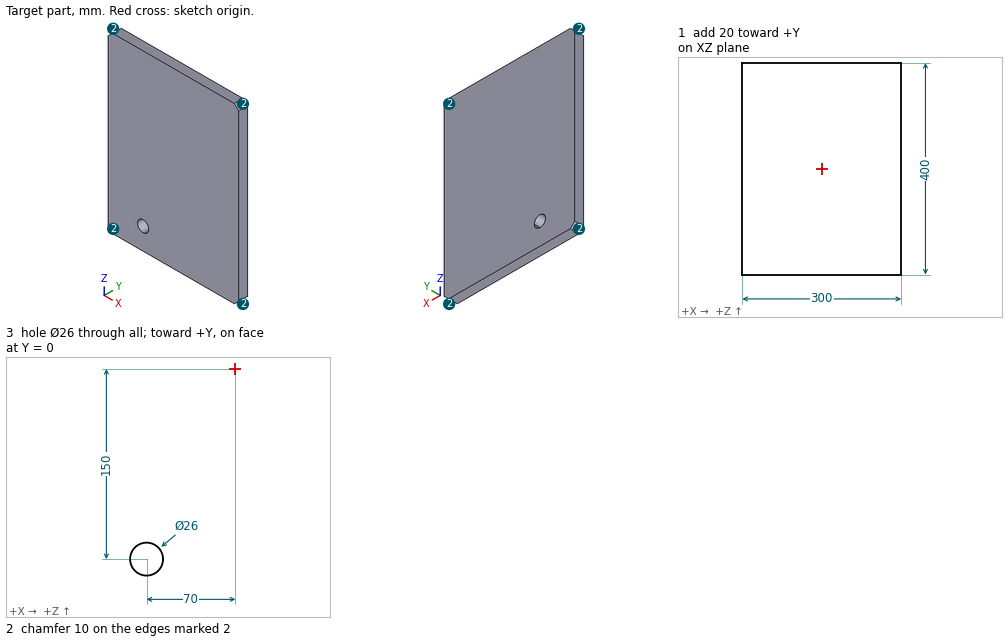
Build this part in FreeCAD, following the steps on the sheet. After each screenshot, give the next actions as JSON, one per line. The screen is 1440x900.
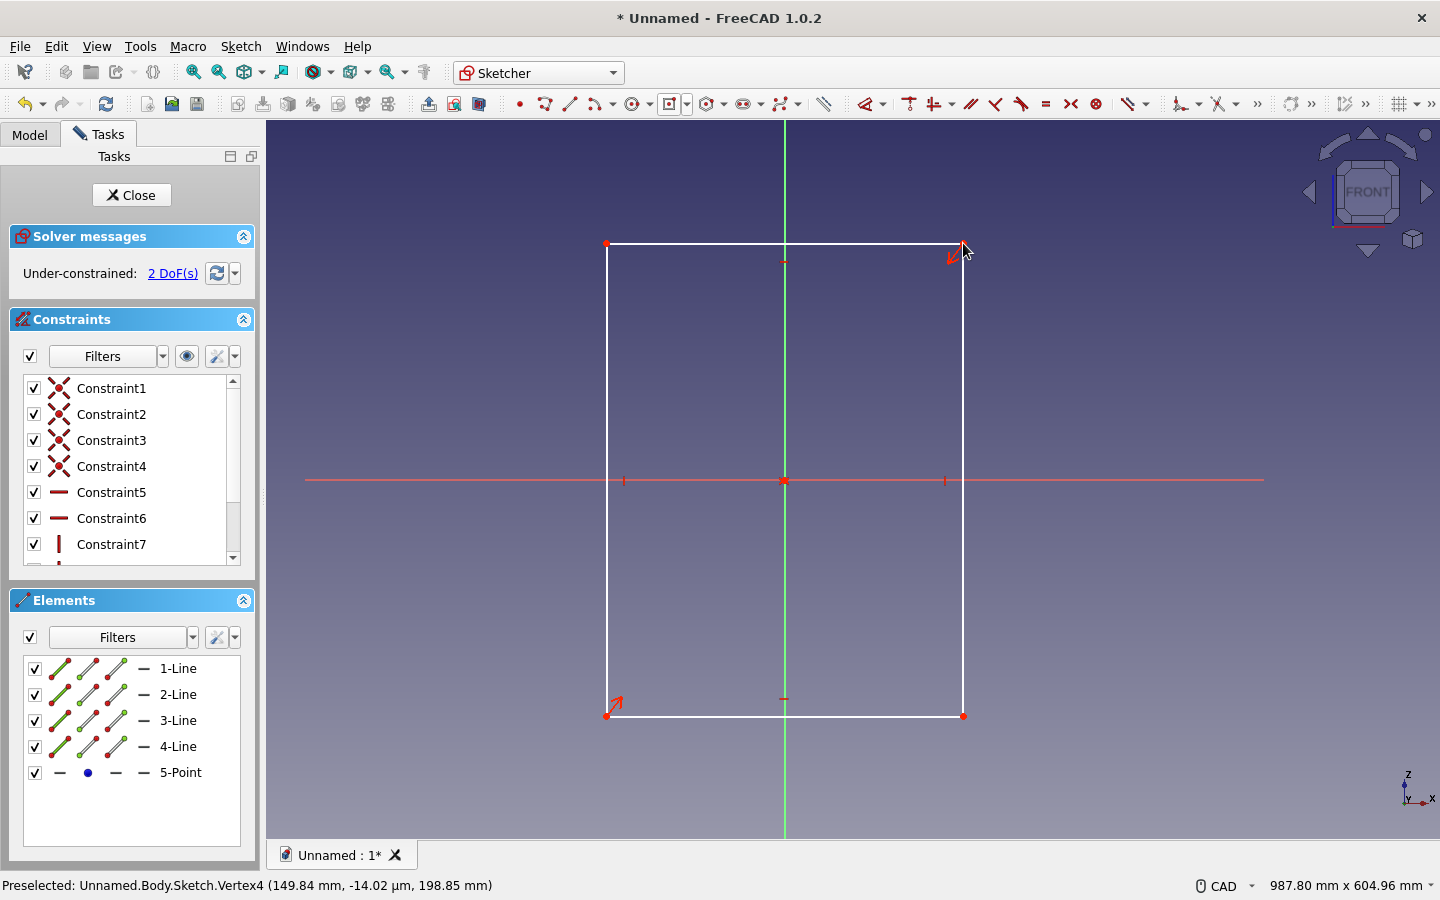
{"action": "left_click", "coordinate": [864, 104]}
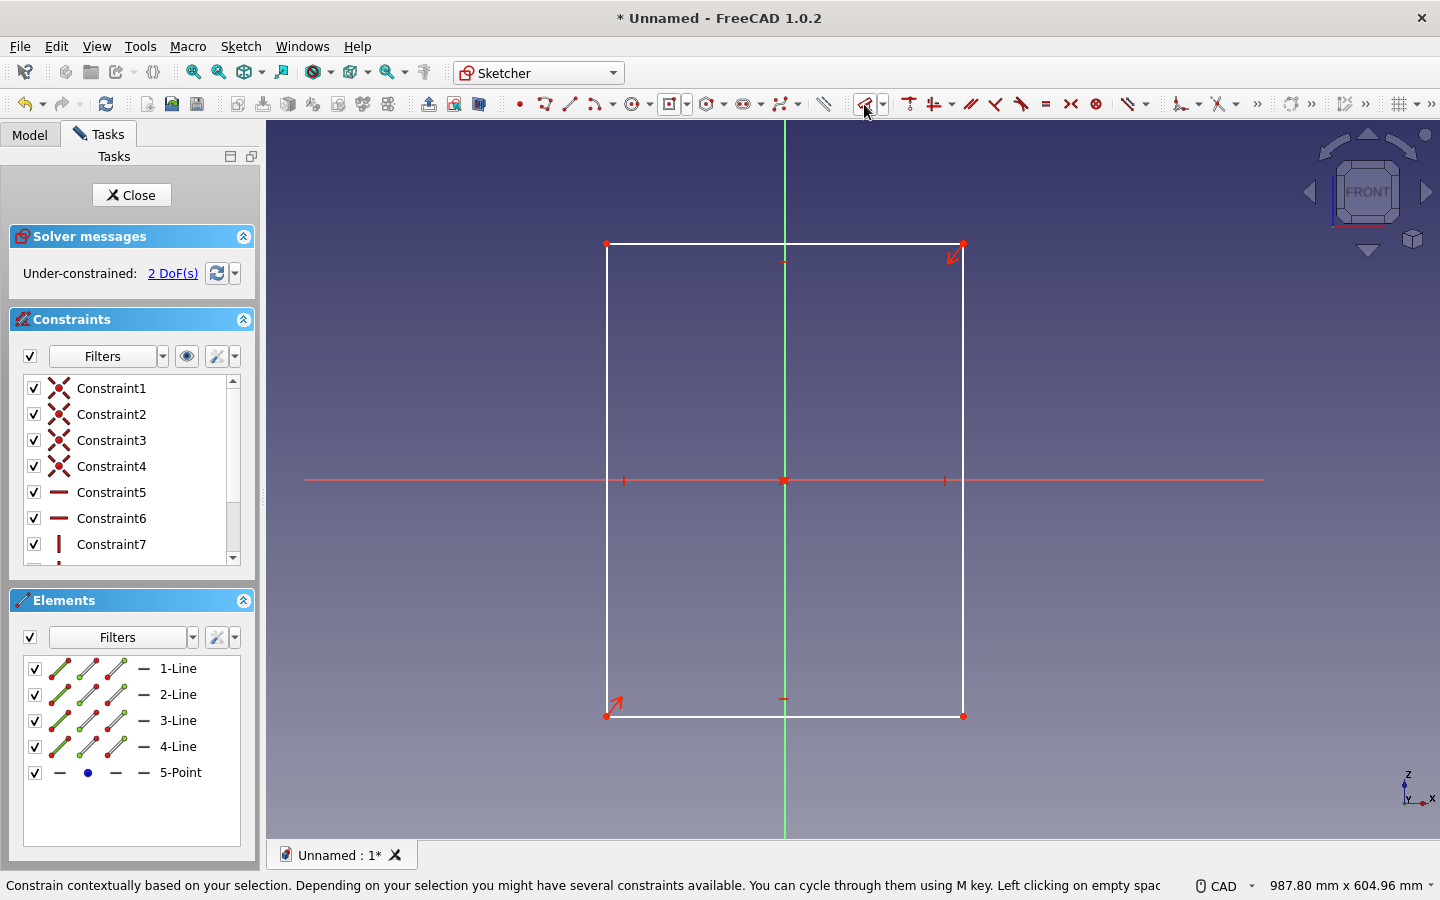
{"action": "left_click", "coordinate": [714, 717]}
{"action": "left_click", "coordinate": [703, 751]}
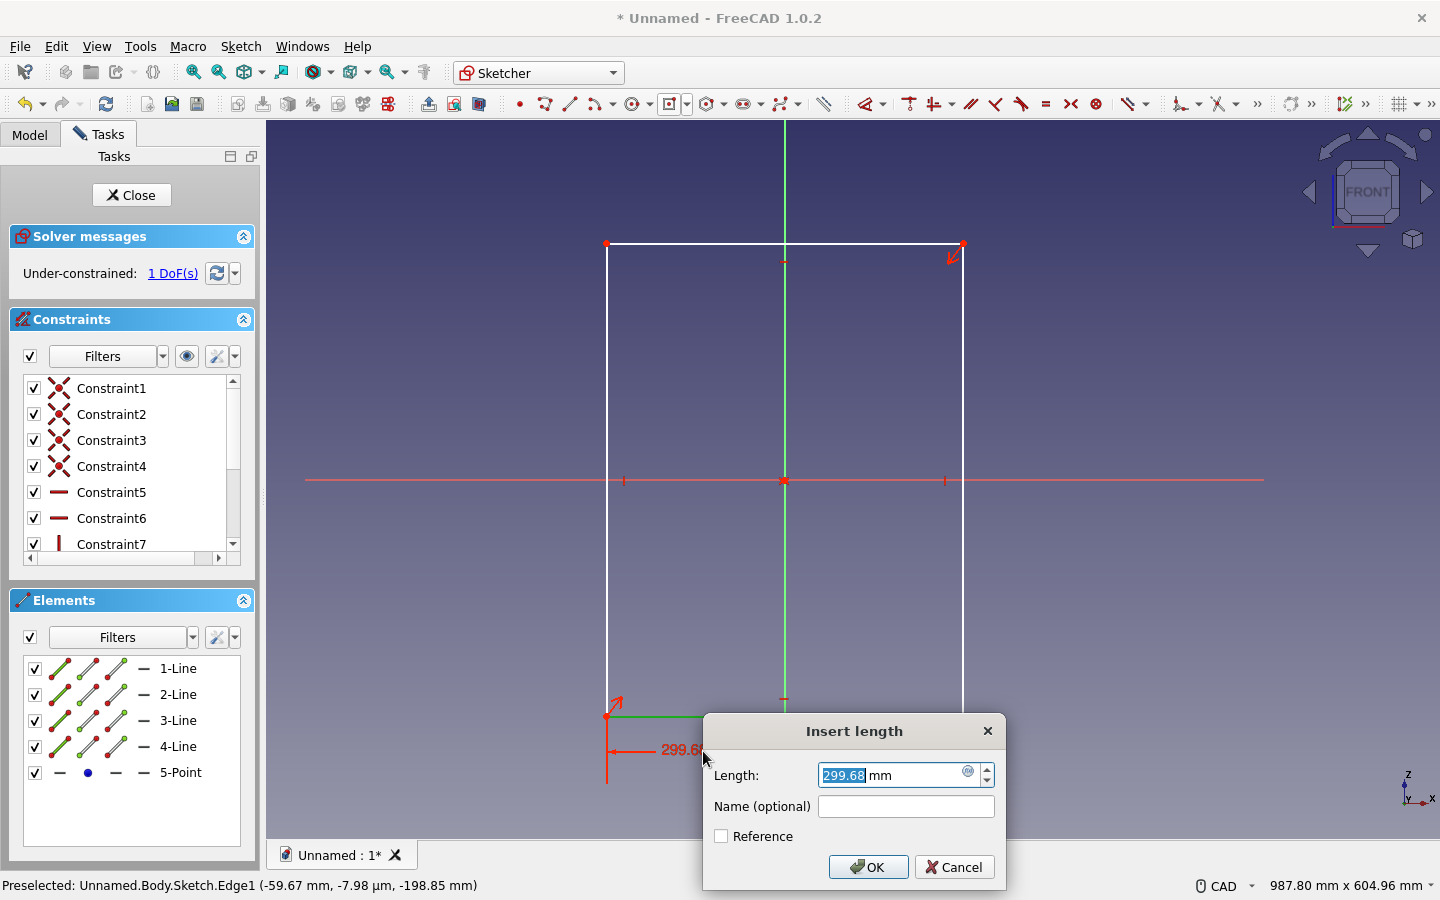
{"action": "type", "text": "300"}
{"action": "key", "text": "Return"}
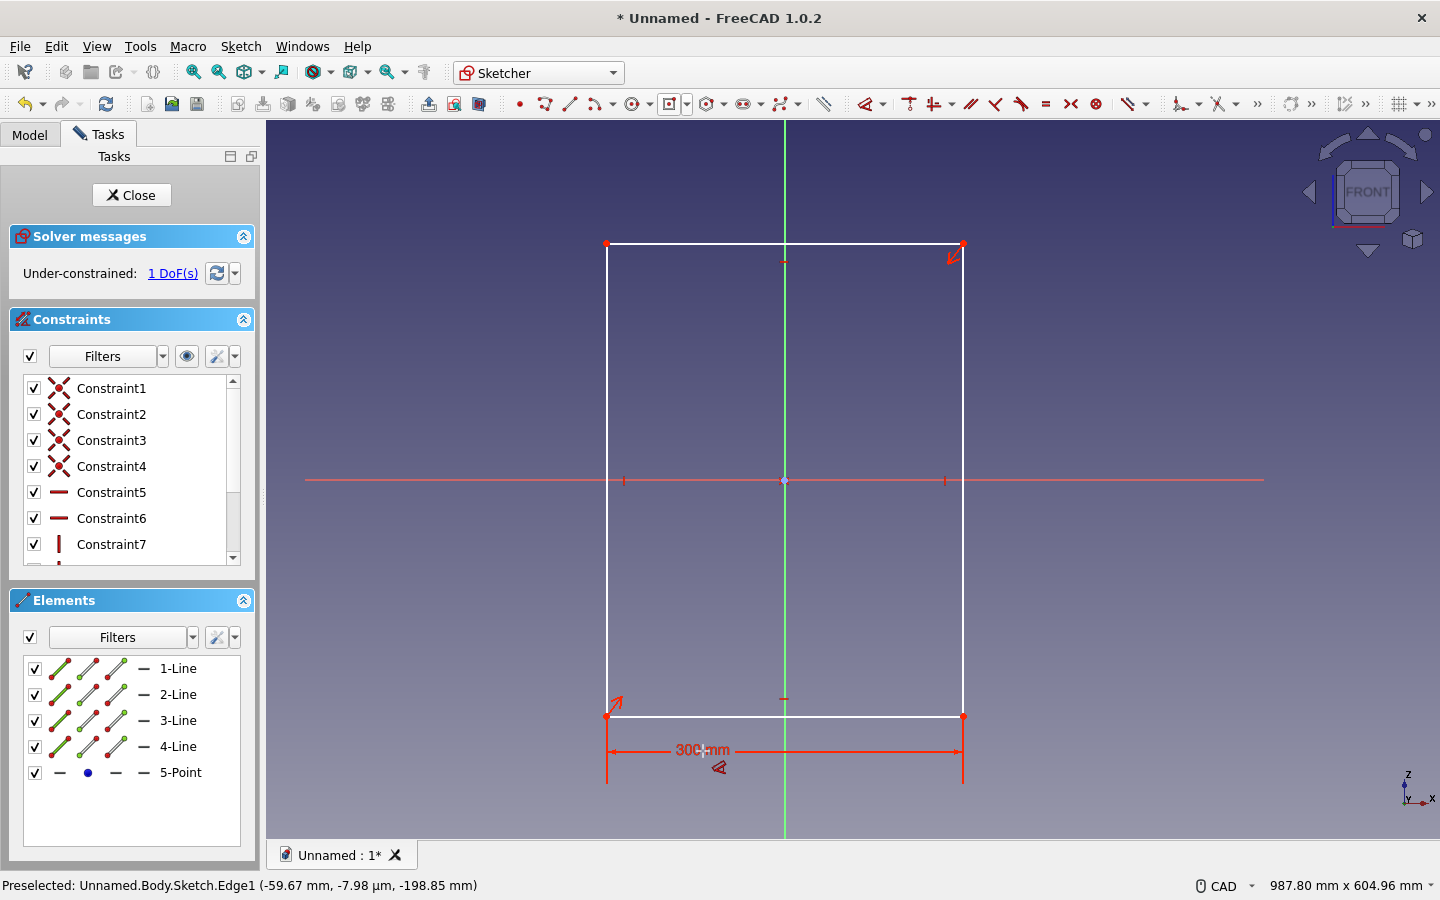
{"action": "left_click", "coordinate": [963, 575]}
{"action": "left_click", "coordinate": [997, 372]}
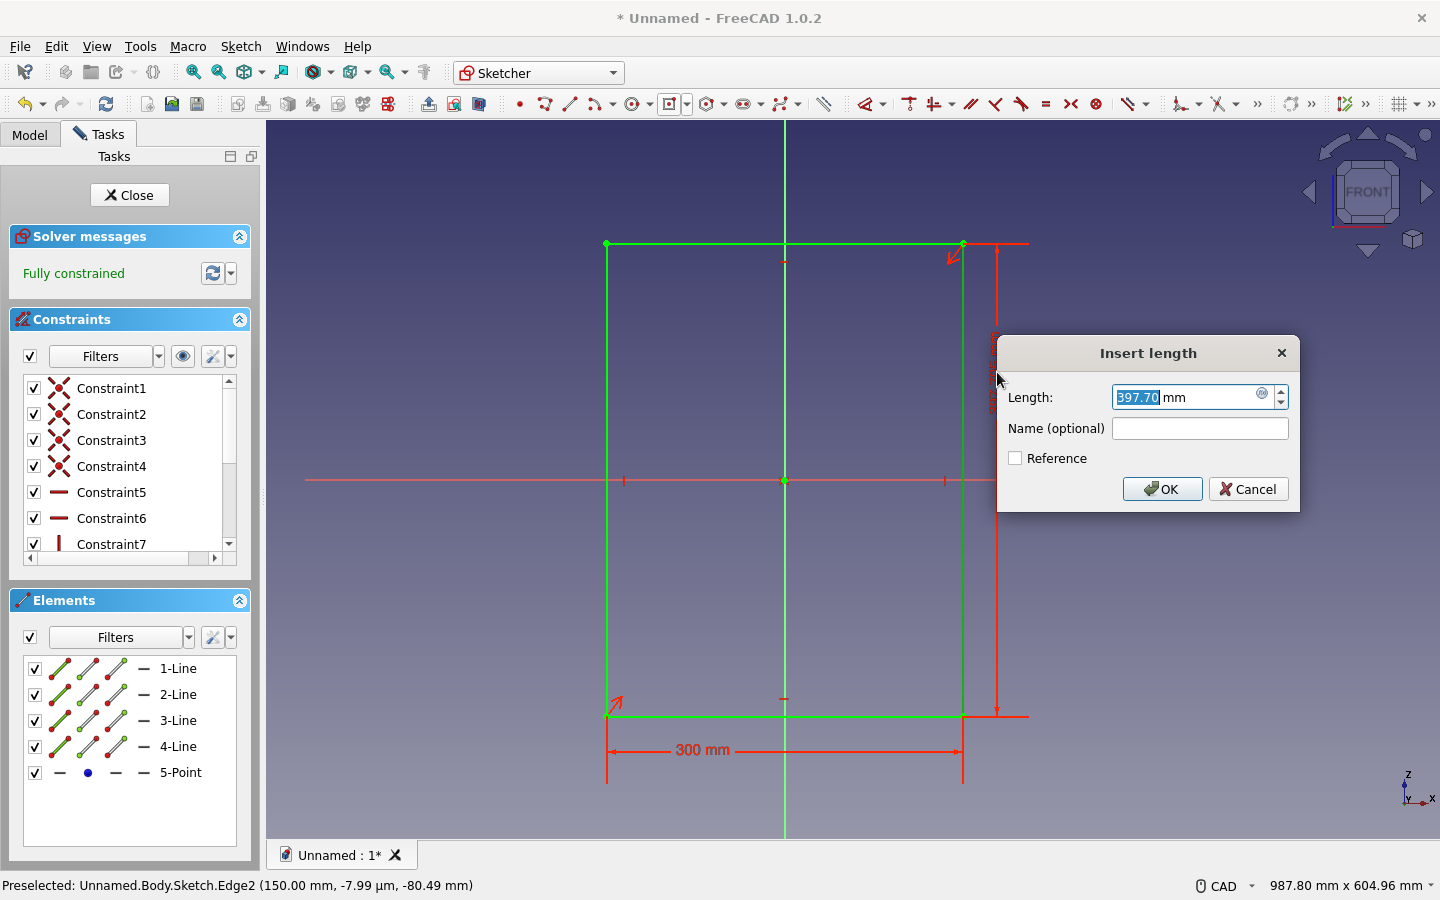
{"action": "type", "text": "400"}
{"action": "key", "text": "Return"}
{"action": "key", "text": "Escape"}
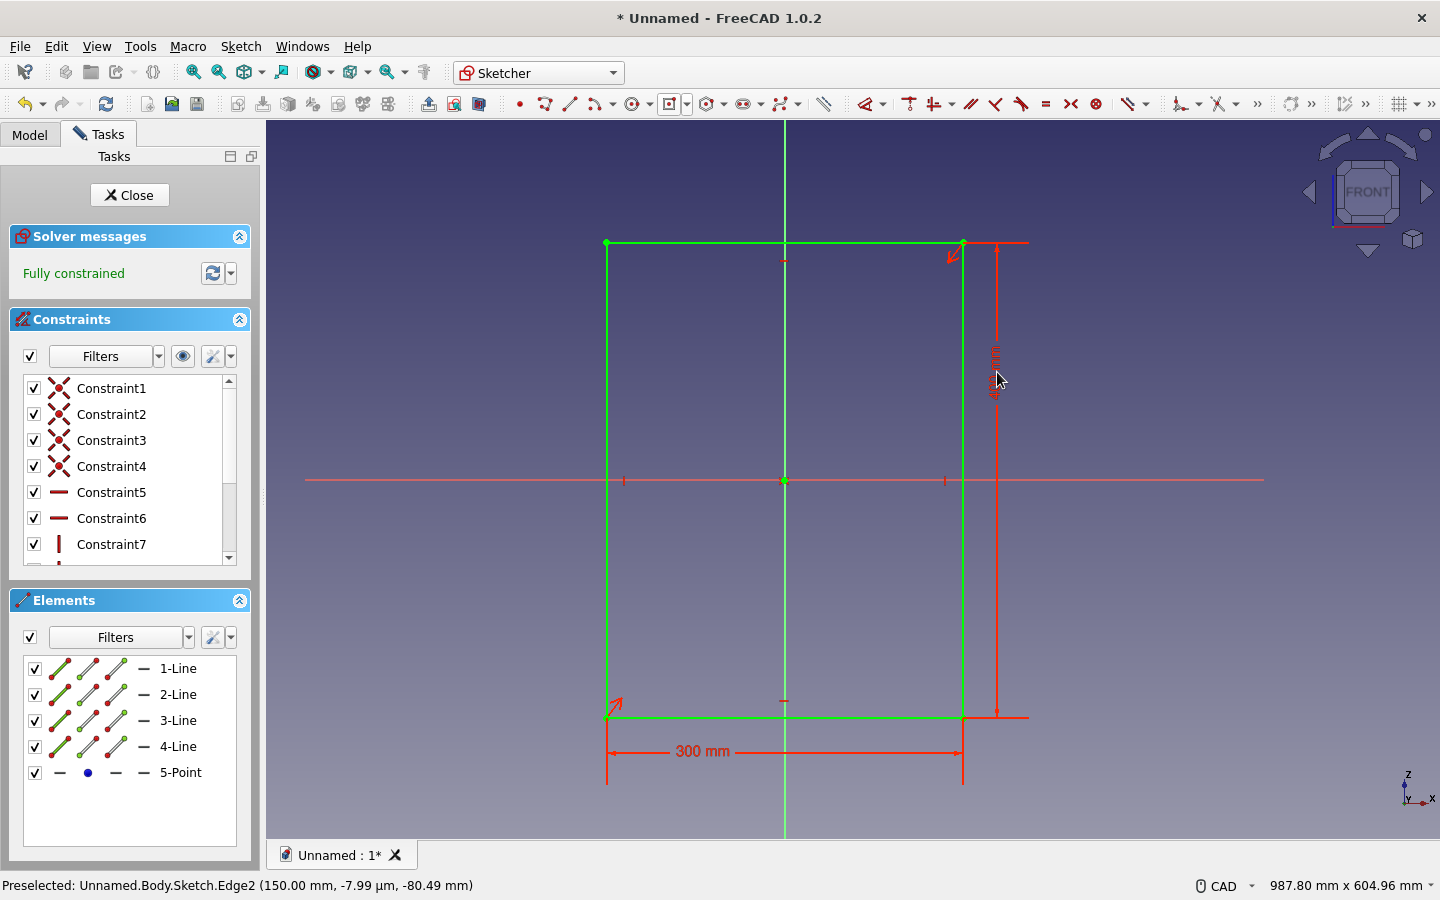
{"action": "left_click", "coordinate": [130, 195]}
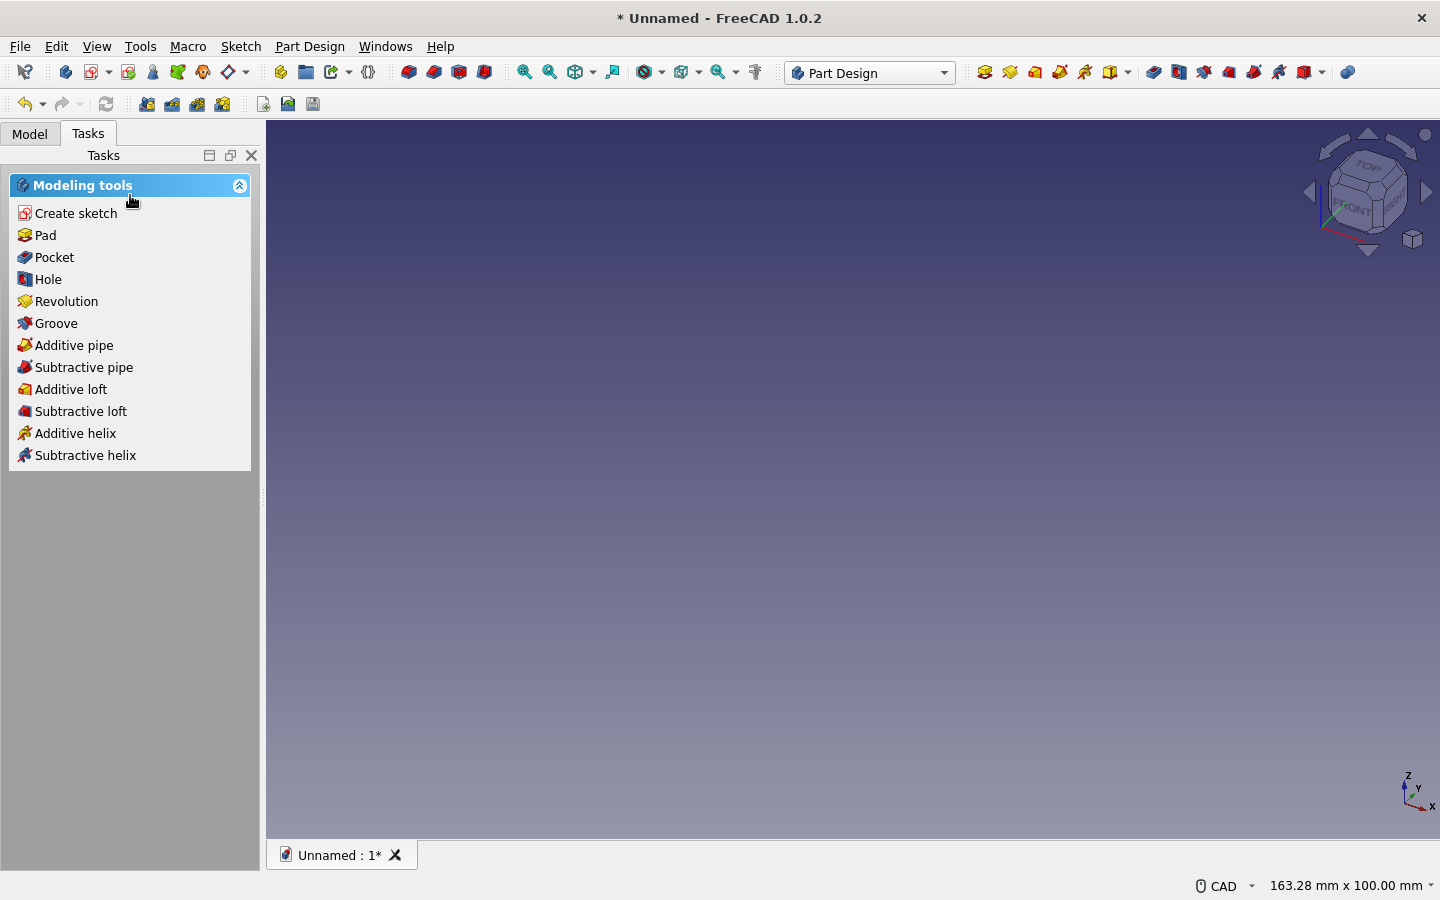
{"action": "left_click", "coordinate": [985, 72]}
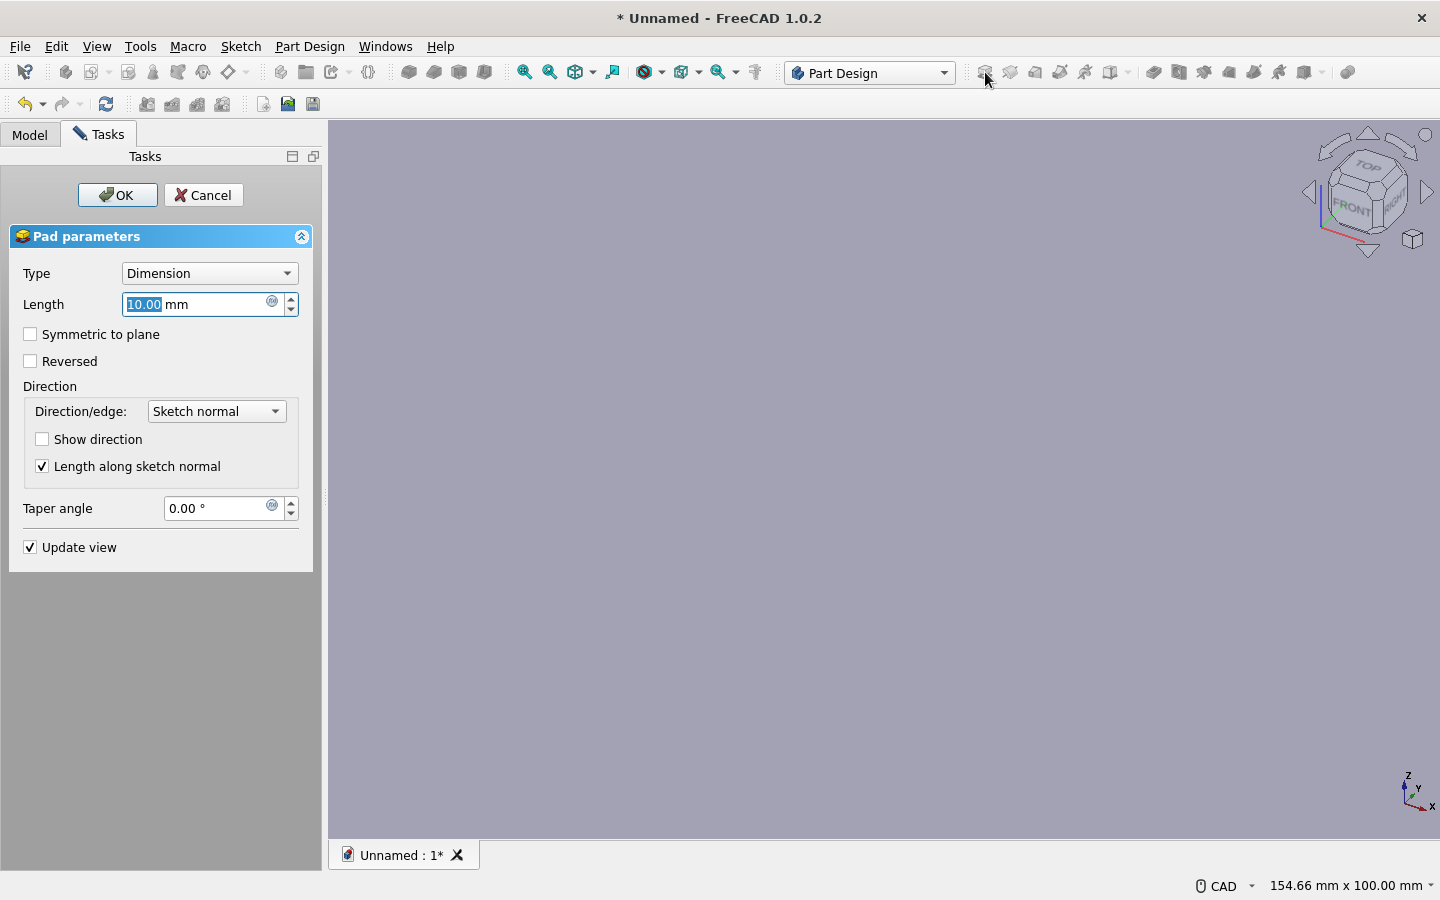
{"action": "type", "text": "20"}
{"action": "key", "text": "Tab"}